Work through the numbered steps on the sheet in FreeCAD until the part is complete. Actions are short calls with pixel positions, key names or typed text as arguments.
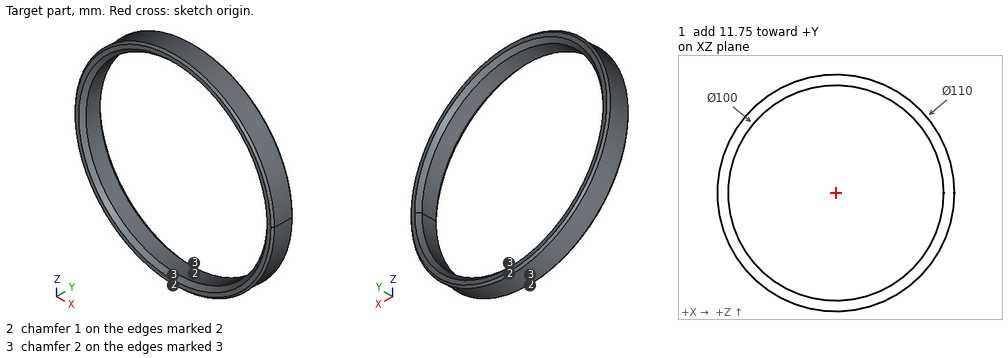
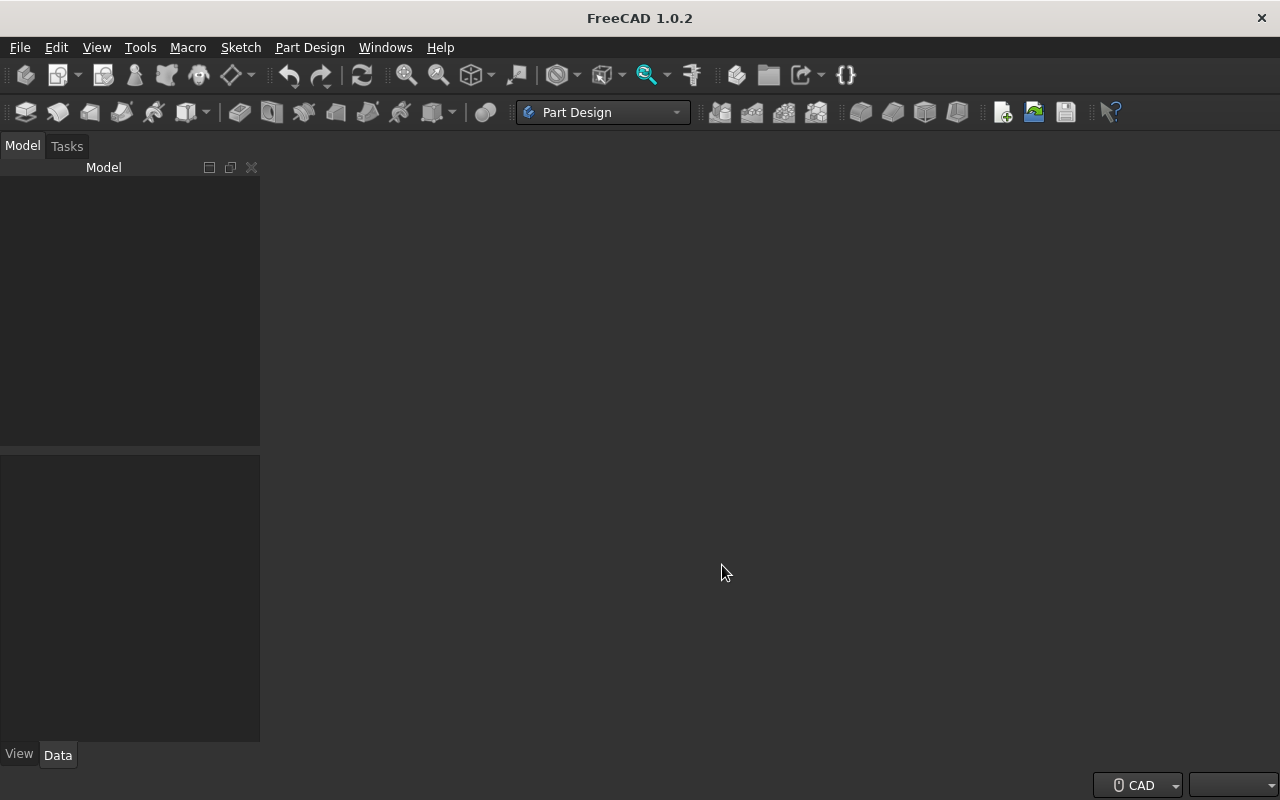
click(1002, 112)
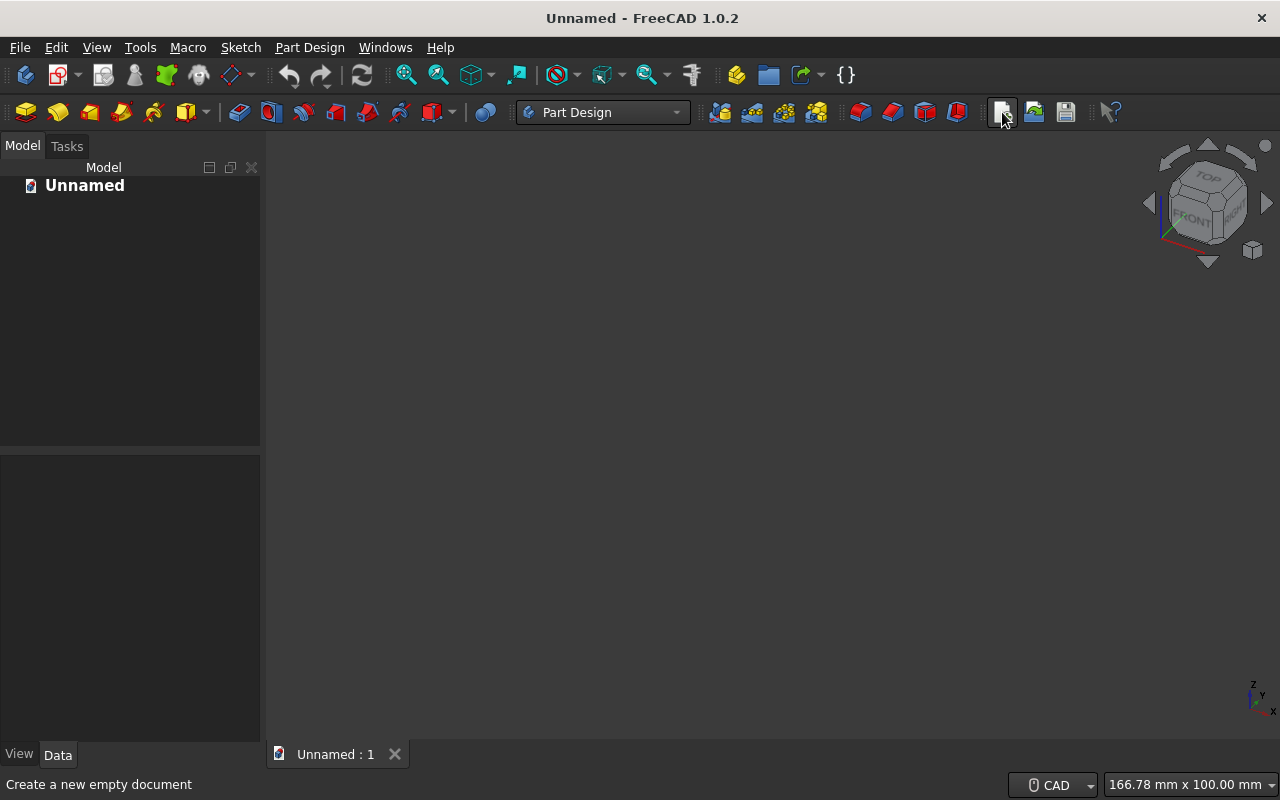
click(58, 76)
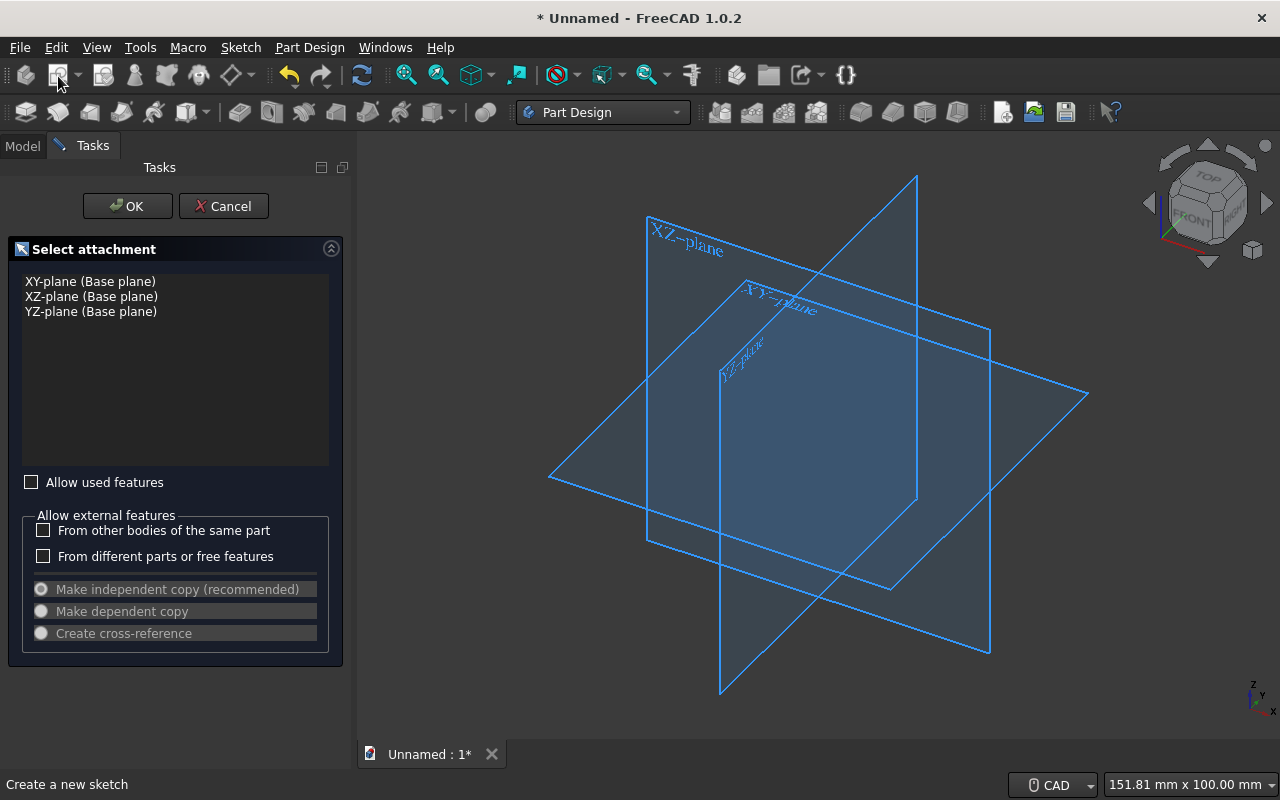
click(82, 296)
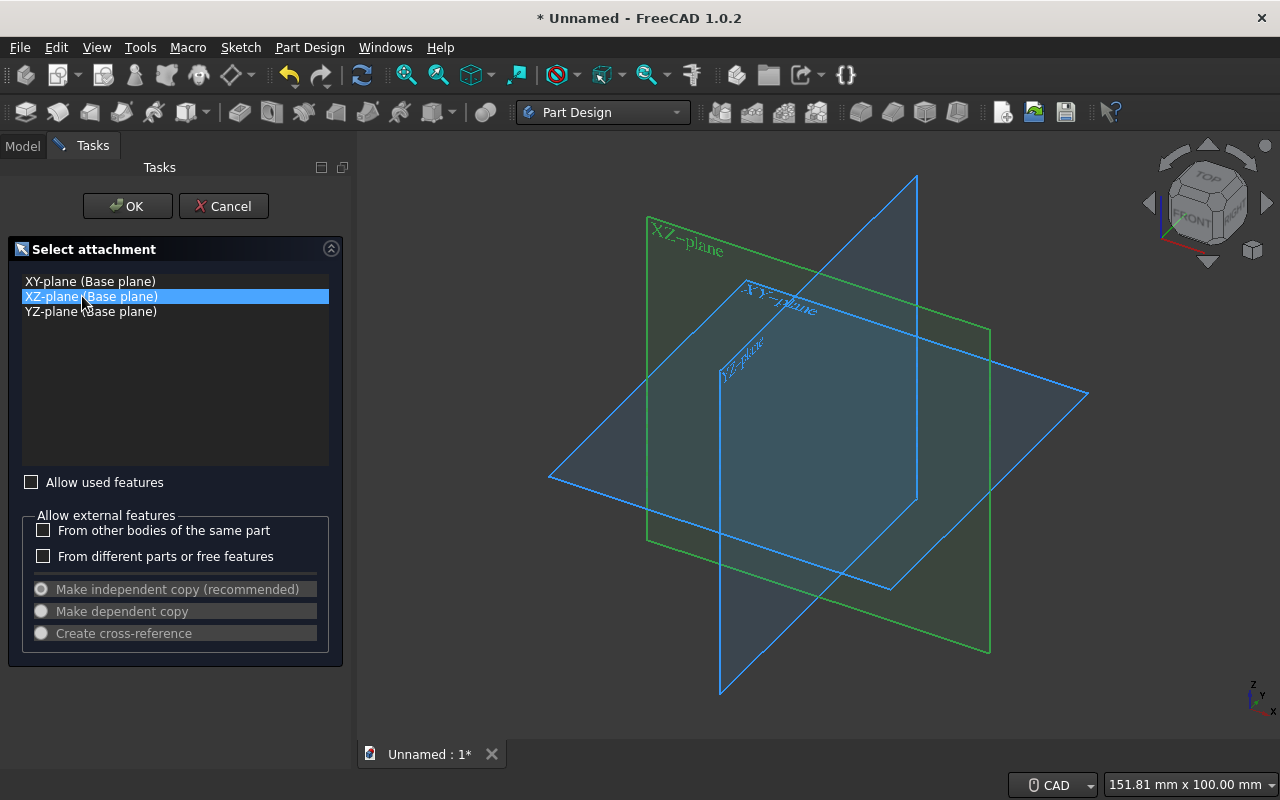
click(128, 206)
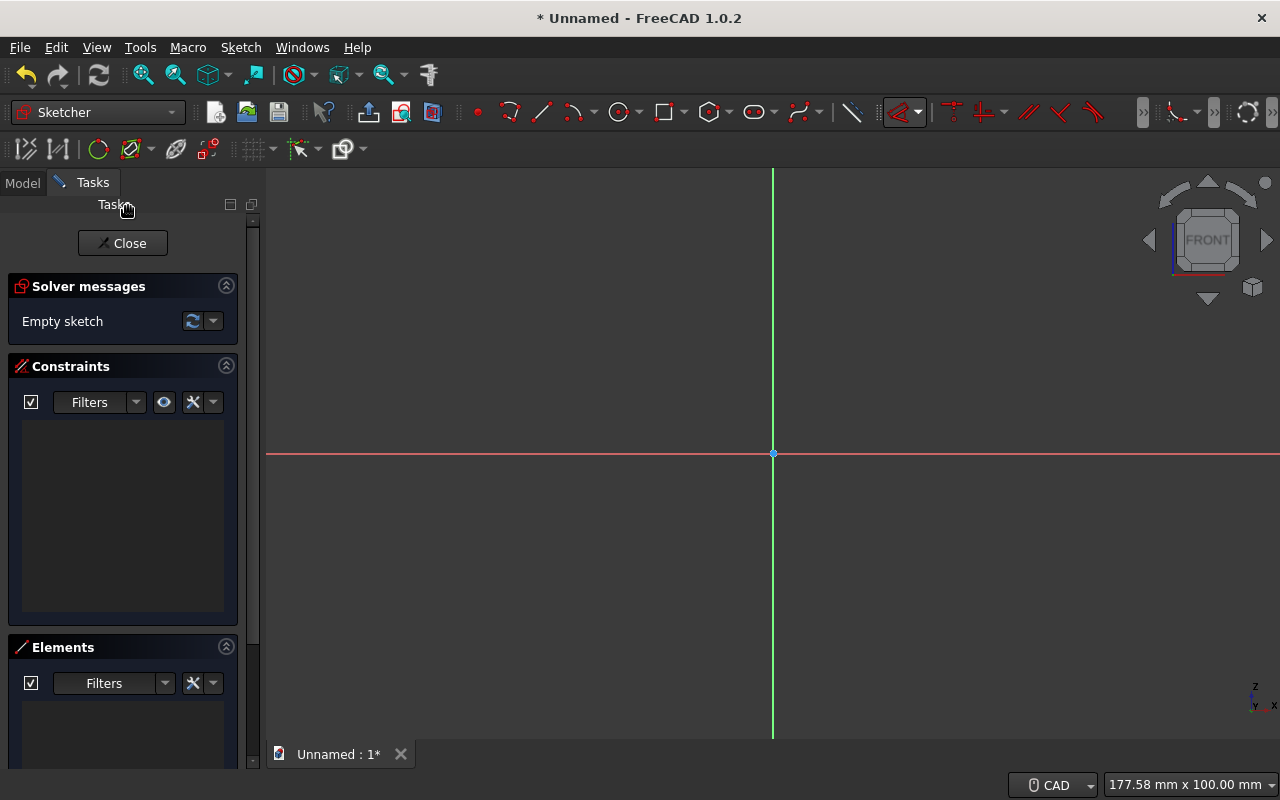
scroll(621, 454, down, 3)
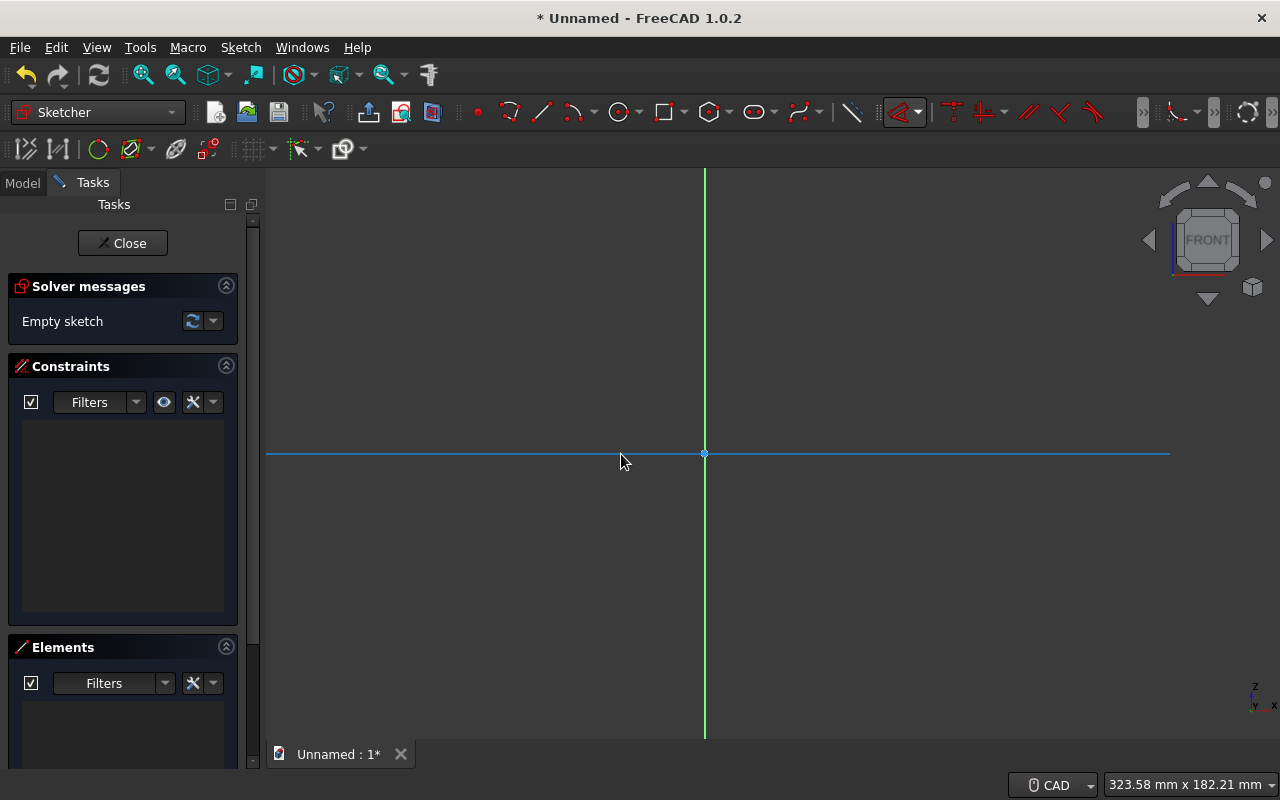
key(g)
key(c)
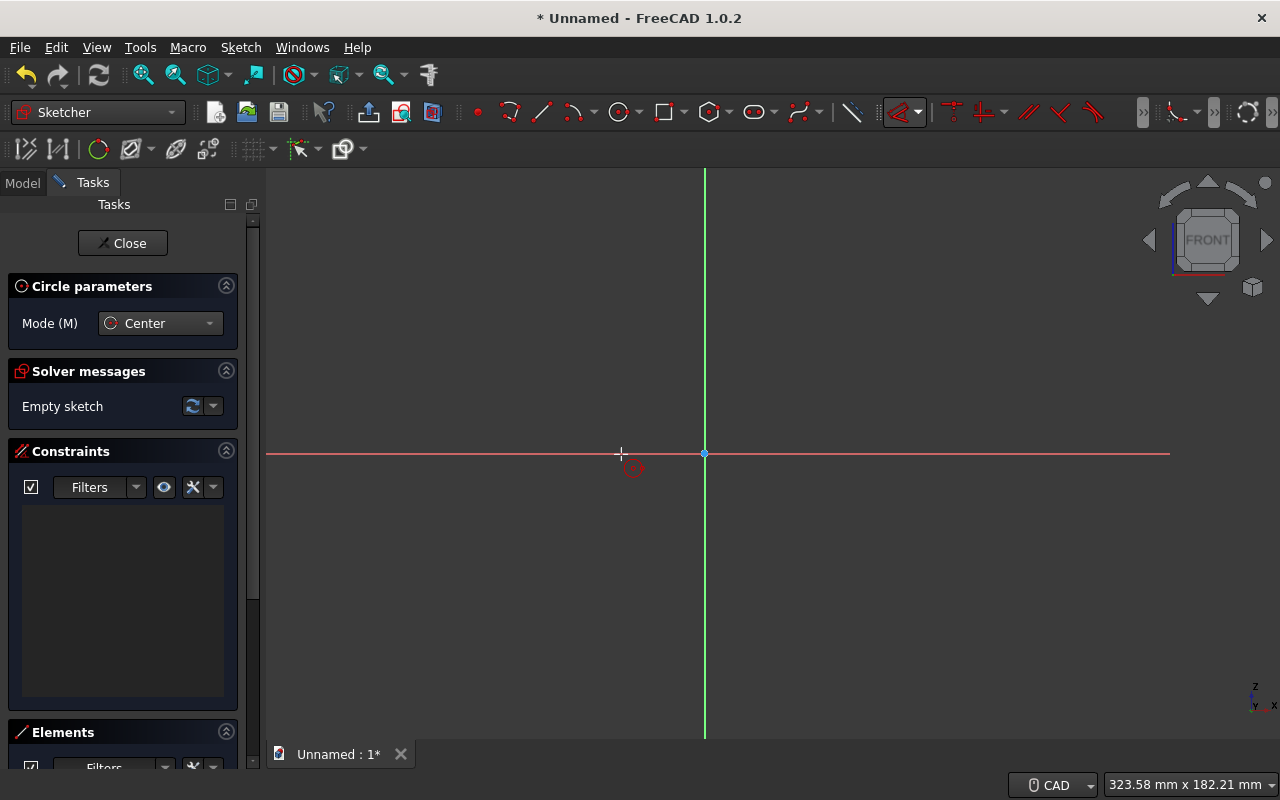
click(705, 454)
move(826, 332)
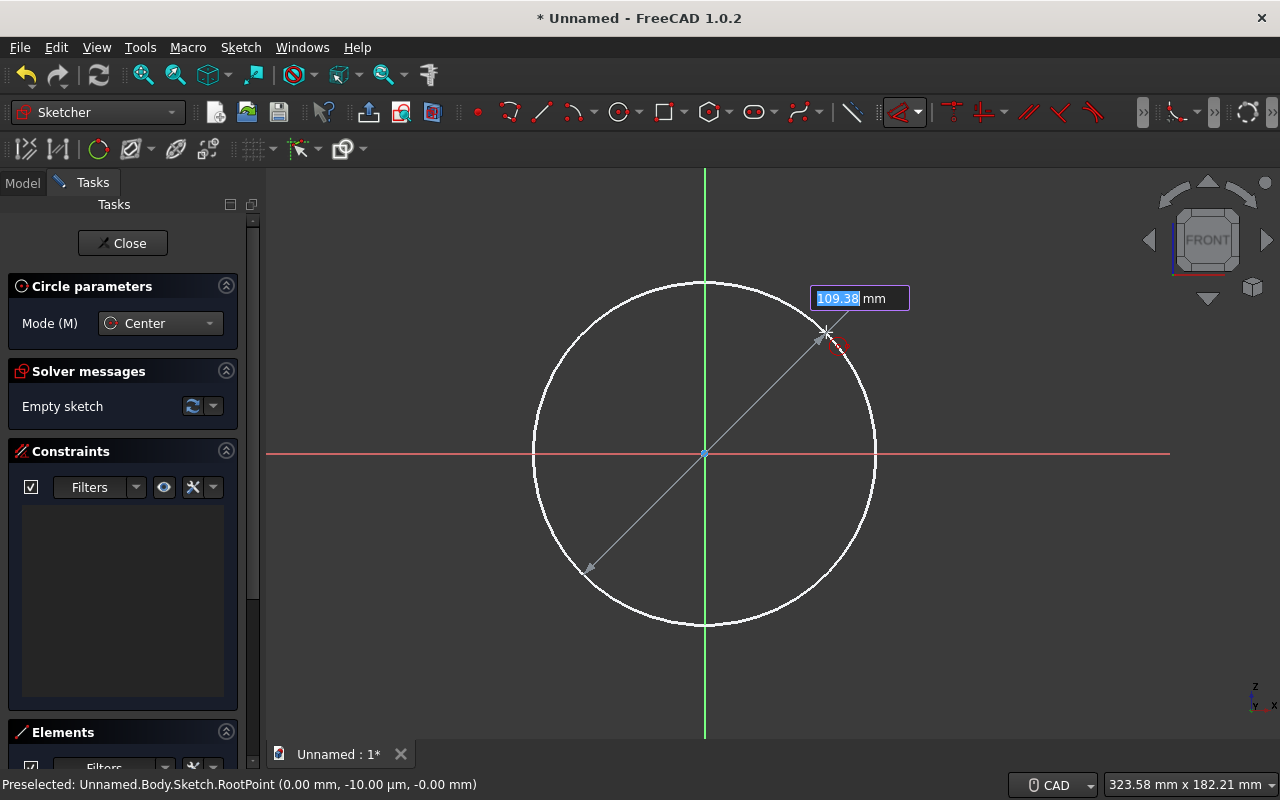
text(110)
key(Return)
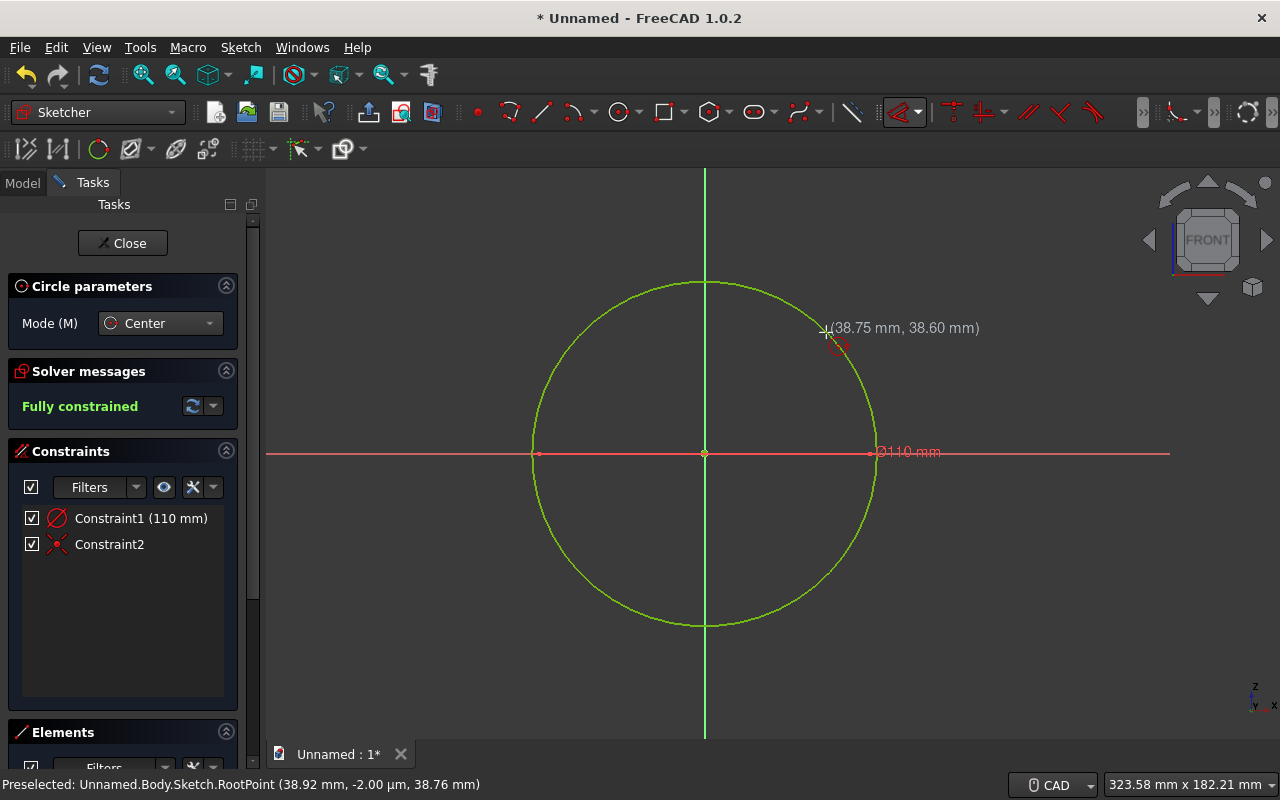
click(705, 454)
move(815, 343)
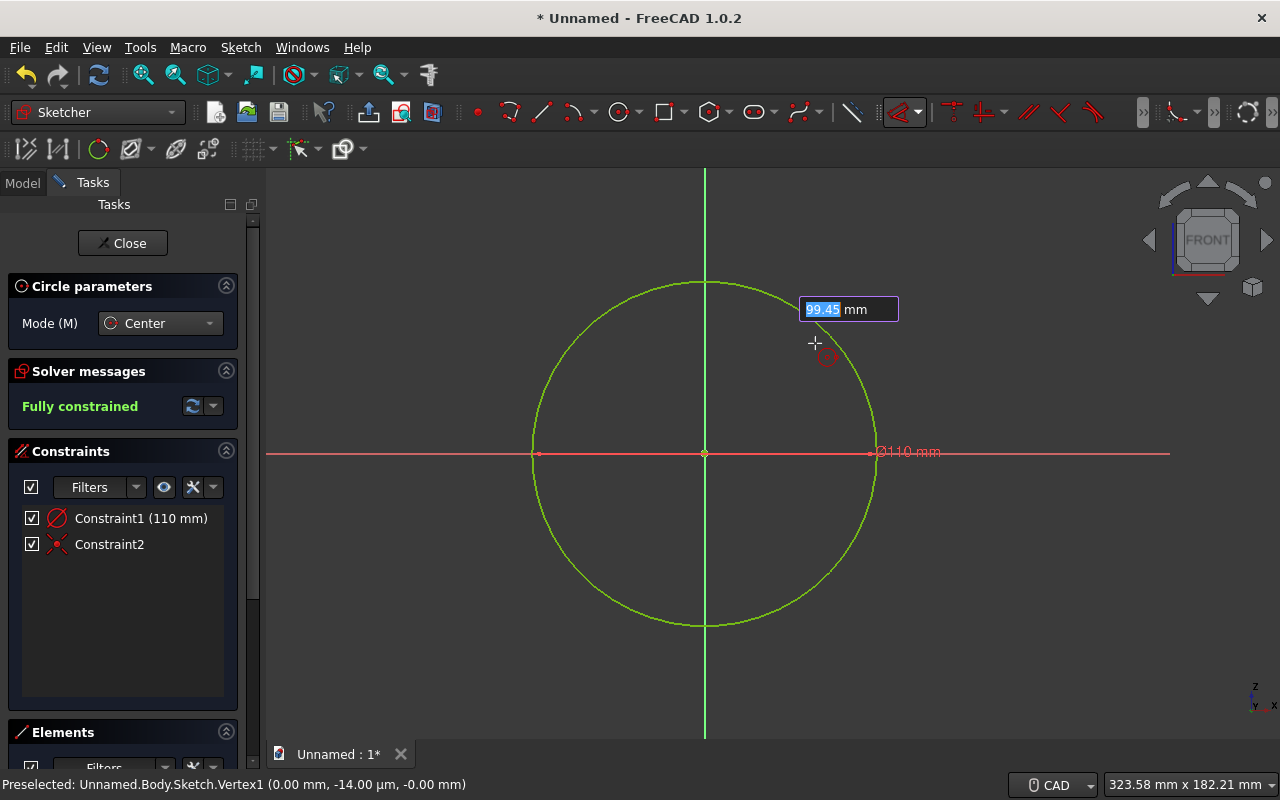
text(100)
key(Return)
key(Escape)